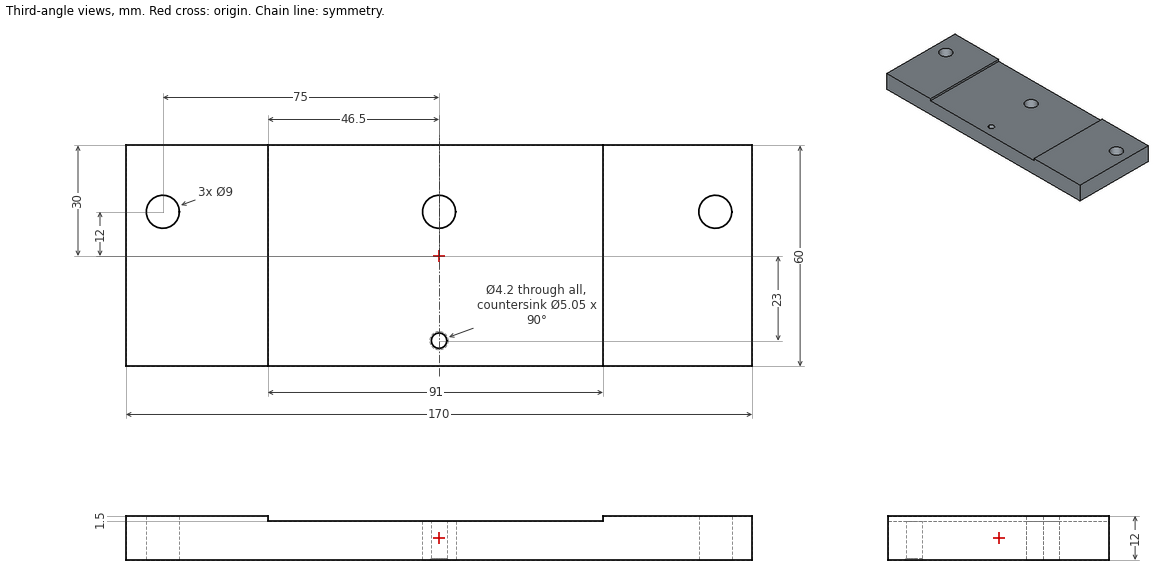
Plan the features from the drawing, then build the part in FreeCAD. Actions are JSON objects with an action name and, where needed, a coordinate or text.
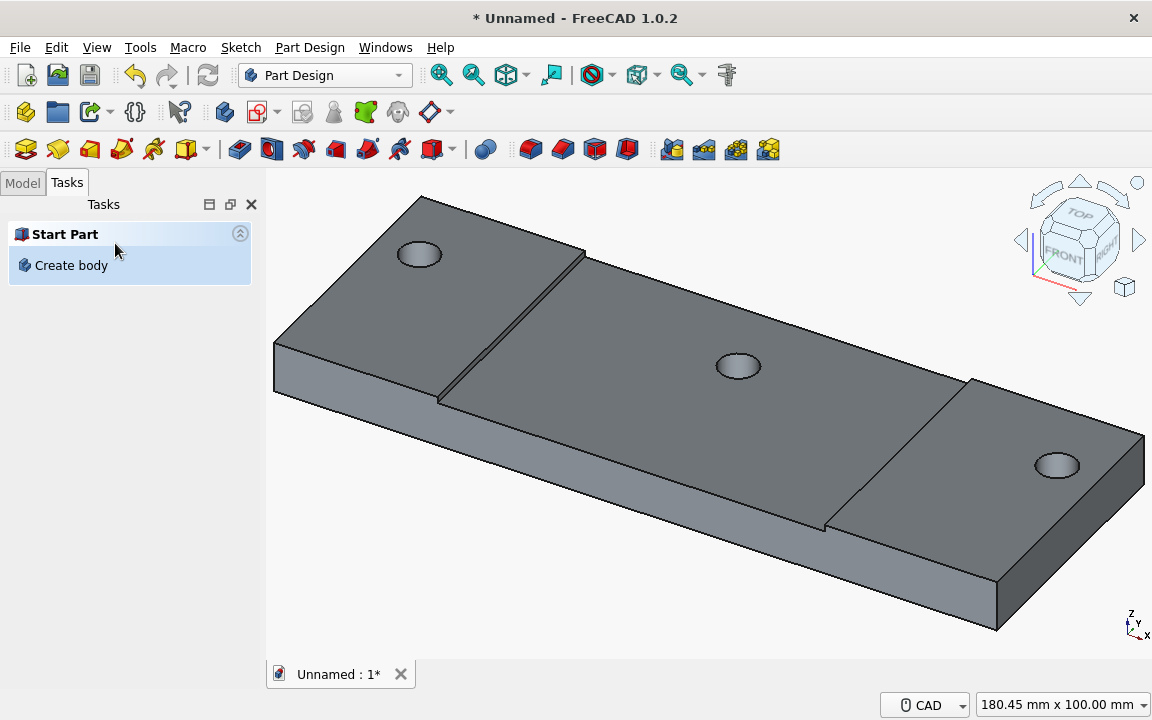
{"action": "key", "text": "5"}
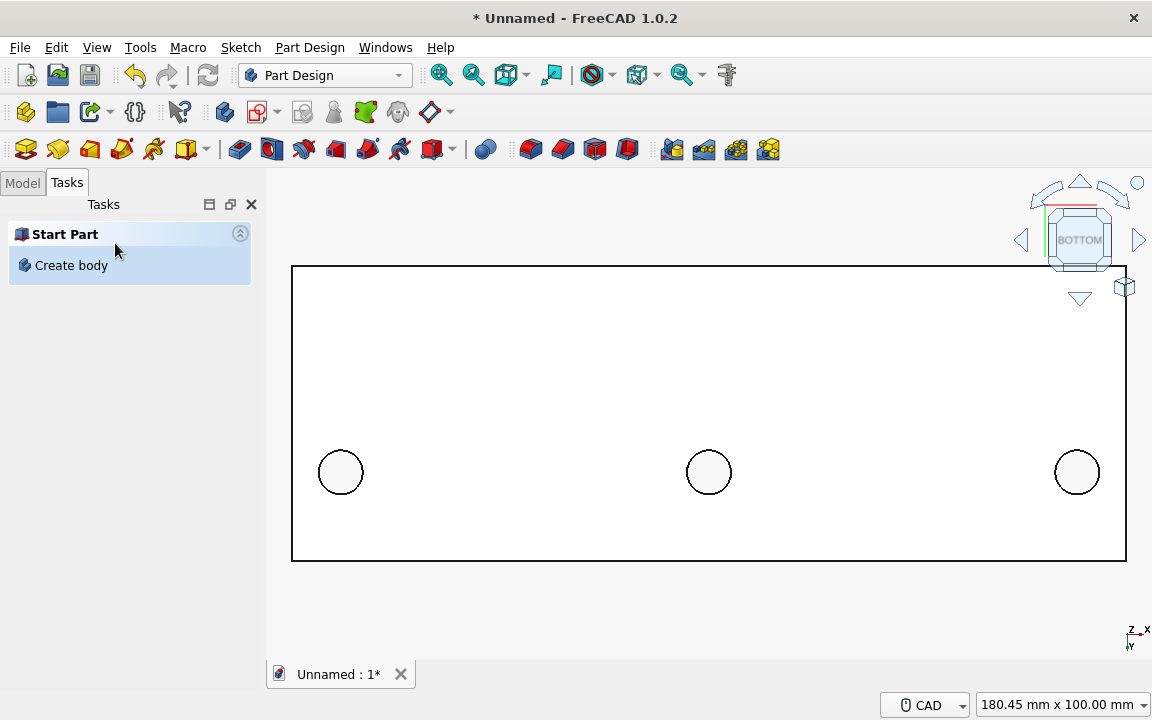
{"action": "left_click", "coordinate": [471, 412]}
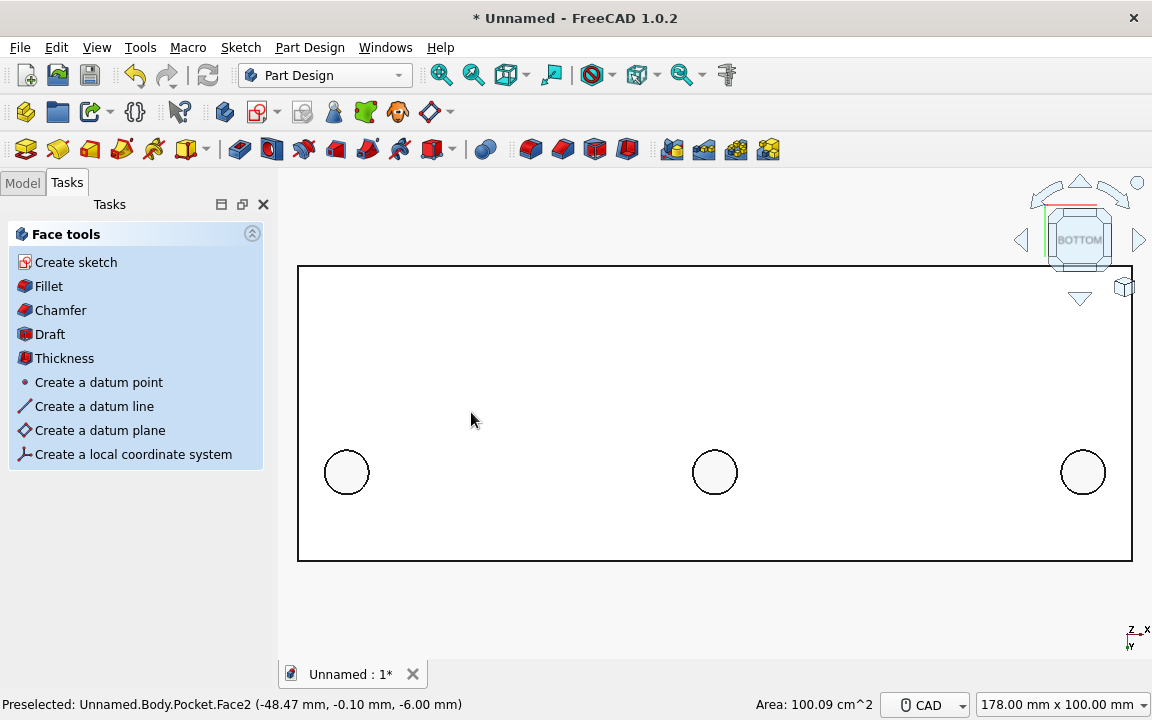
{"action": "left_click", "coordinate": [258, 112]}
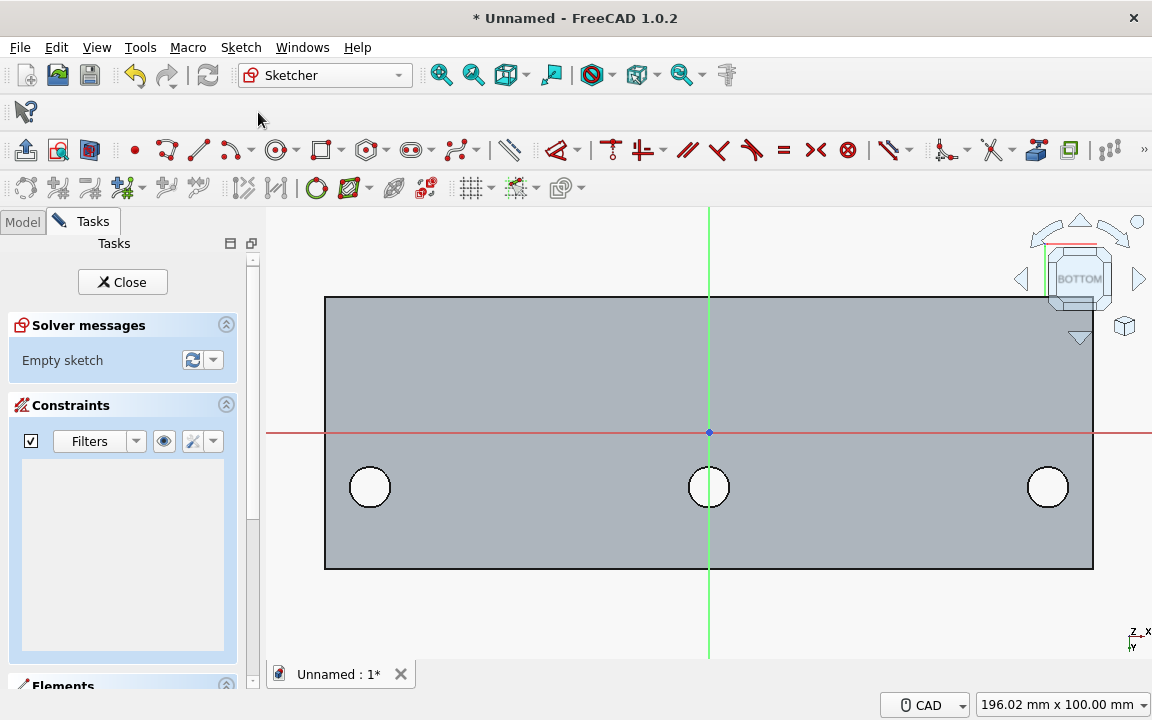
{"action": "scroll", "coordinate": [714, 321], "scroll_direction": "up", "scroll_amount": 13}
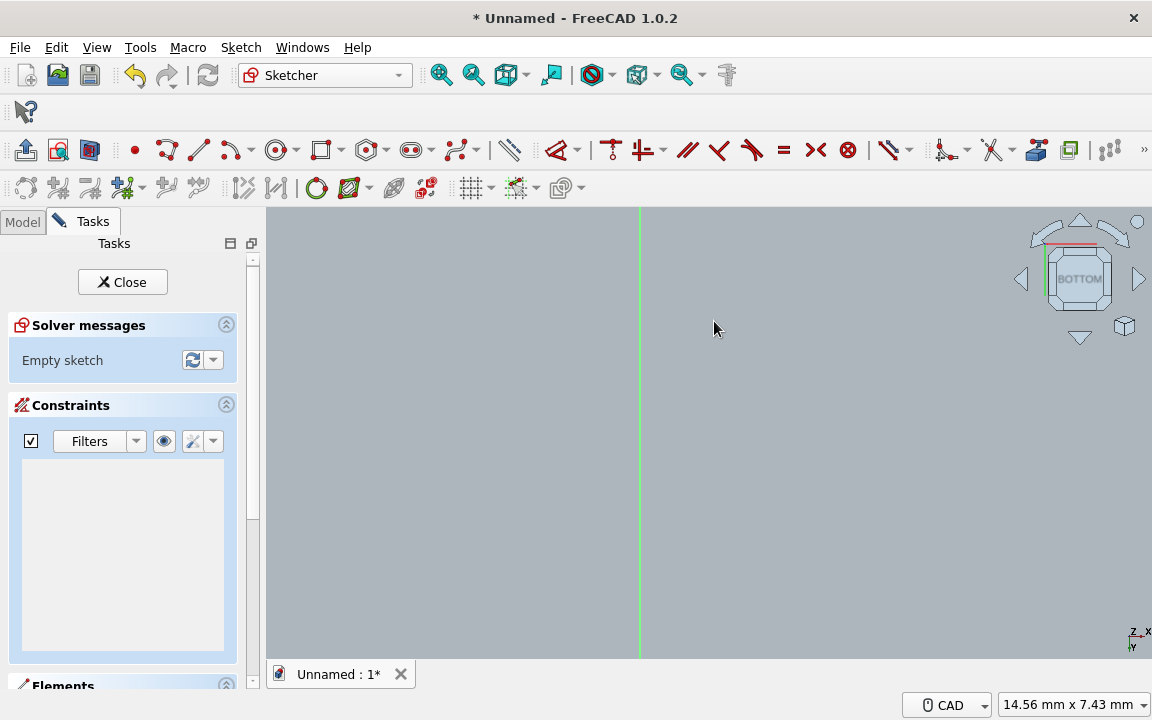
{"action": "key", "text": "g c"}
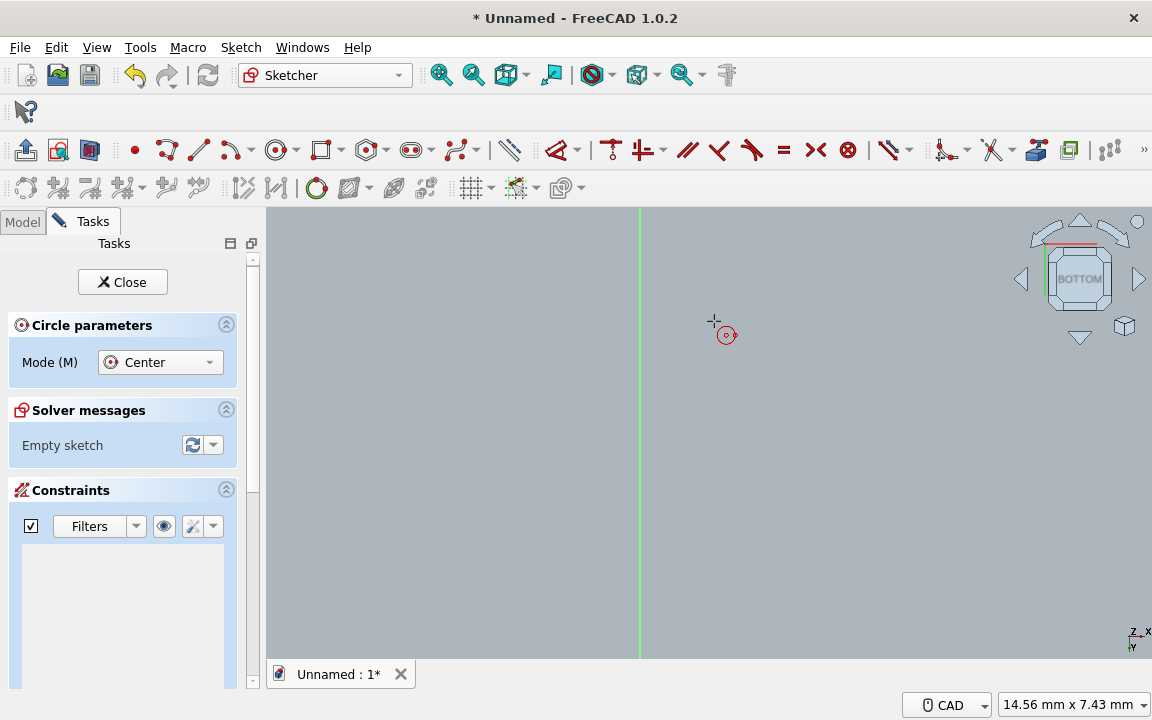
{"action": "left_click", "coordinate": [640, 426]}
{"action": "left_click", "coordinate": [731, 336]}
{"action": "key", "text": "Escape"}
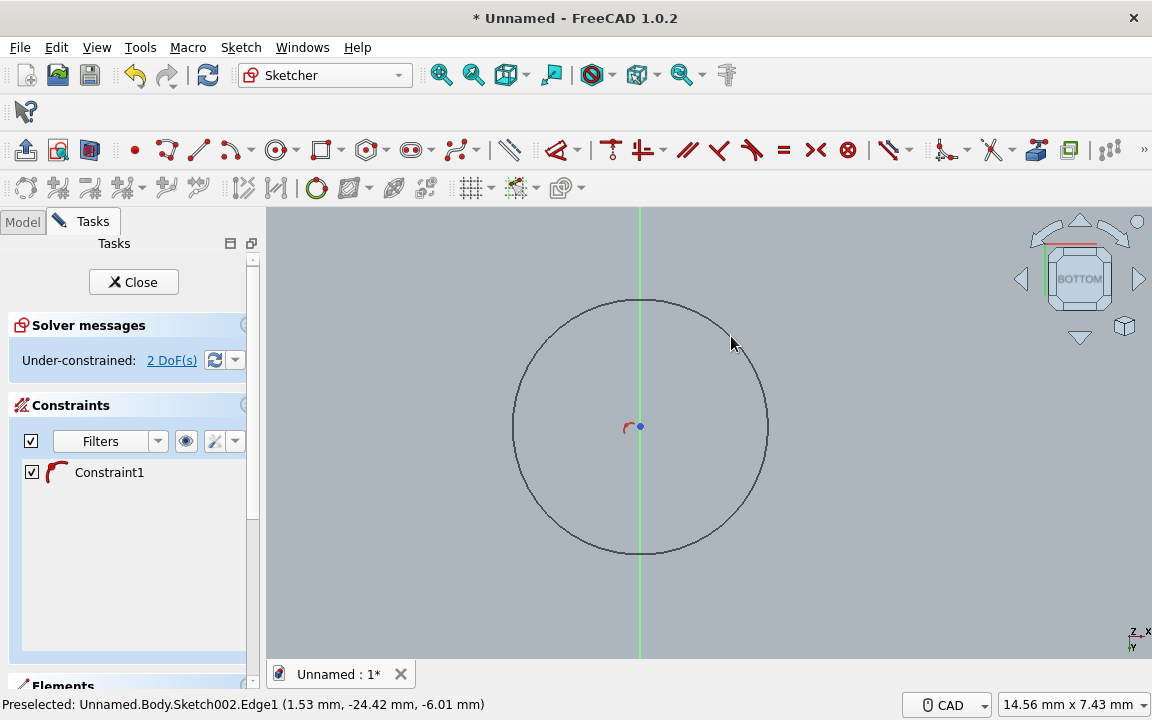
{"action": "key", "text": "d"}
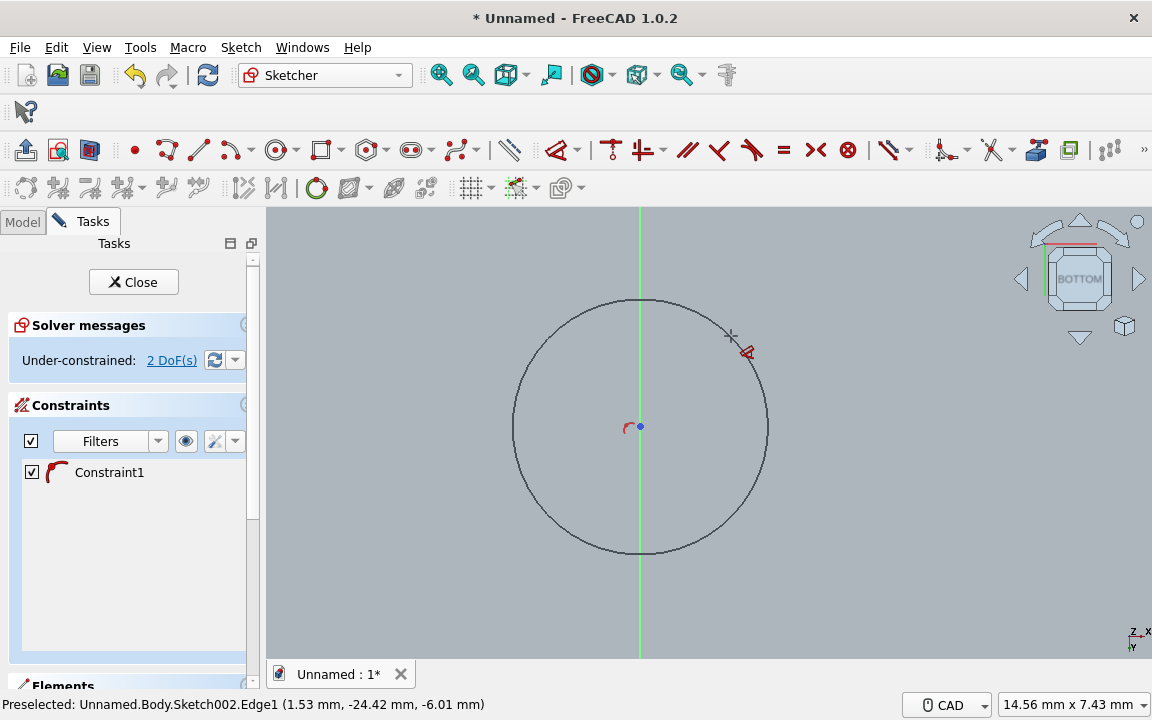
{"action": "left_click", "coordinate": [730, 336]}
{"action": "left_click", "coordinate": [752, 313]}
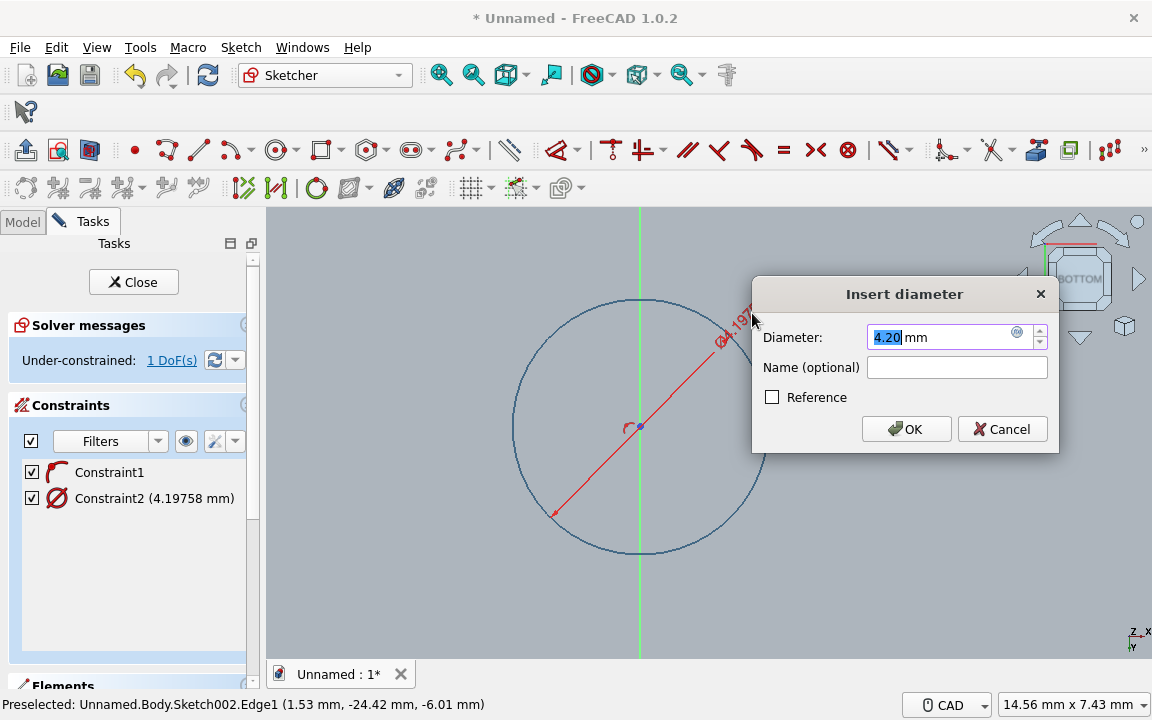
{"action": "type", "text": "4.2"}
{"action": "key", "text": "Return"}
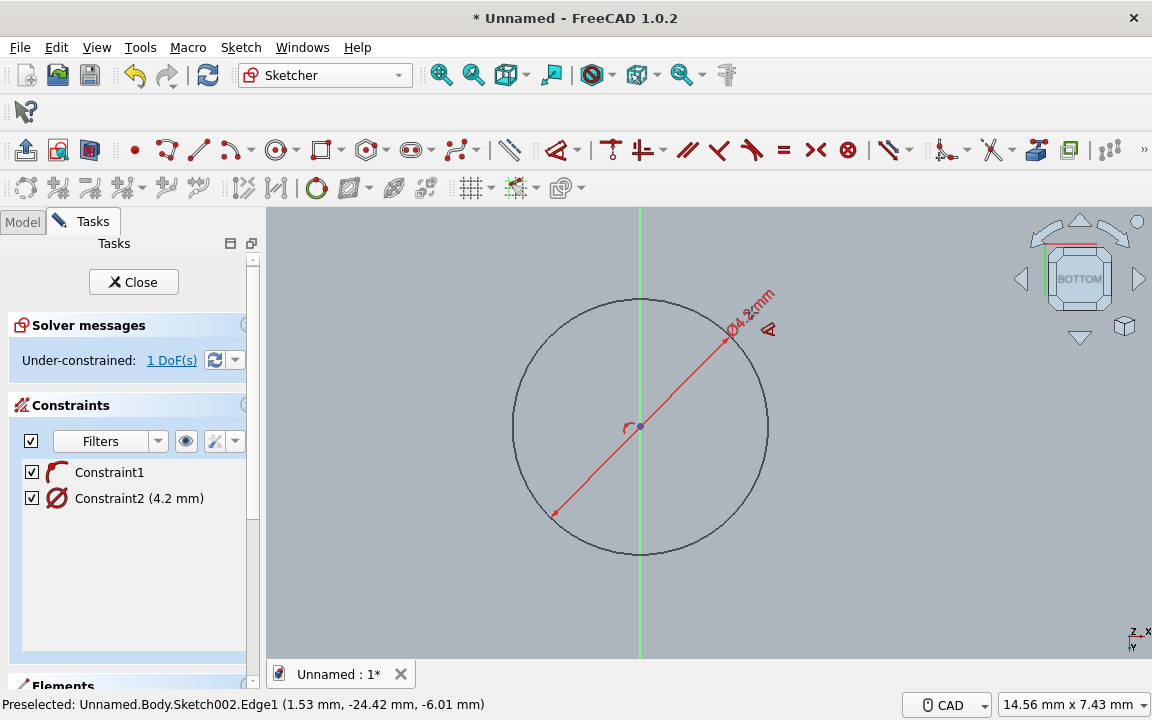
{"action": "left_click", "coordinate": [640, 427]}
{"action": "left_click", "coordinate": [674, 529]}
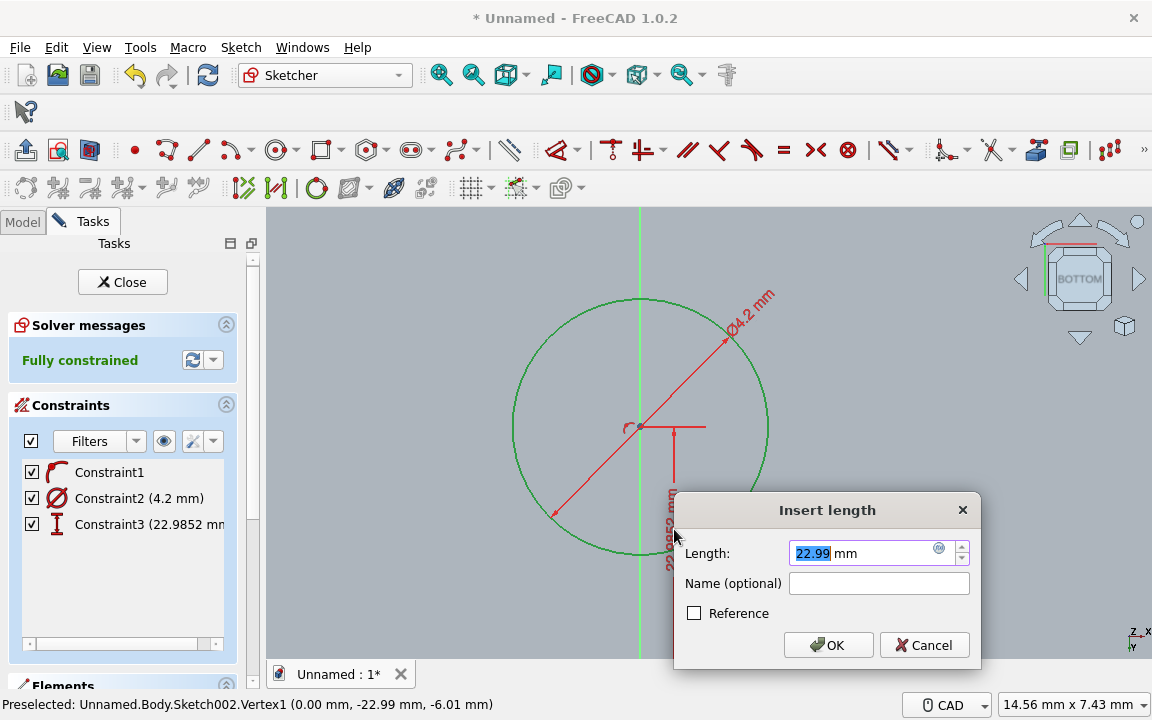
{"action": "type", "text": "23"}
{"action": "key", "text": "Return"}
{"action": "key", "text": "Escape"}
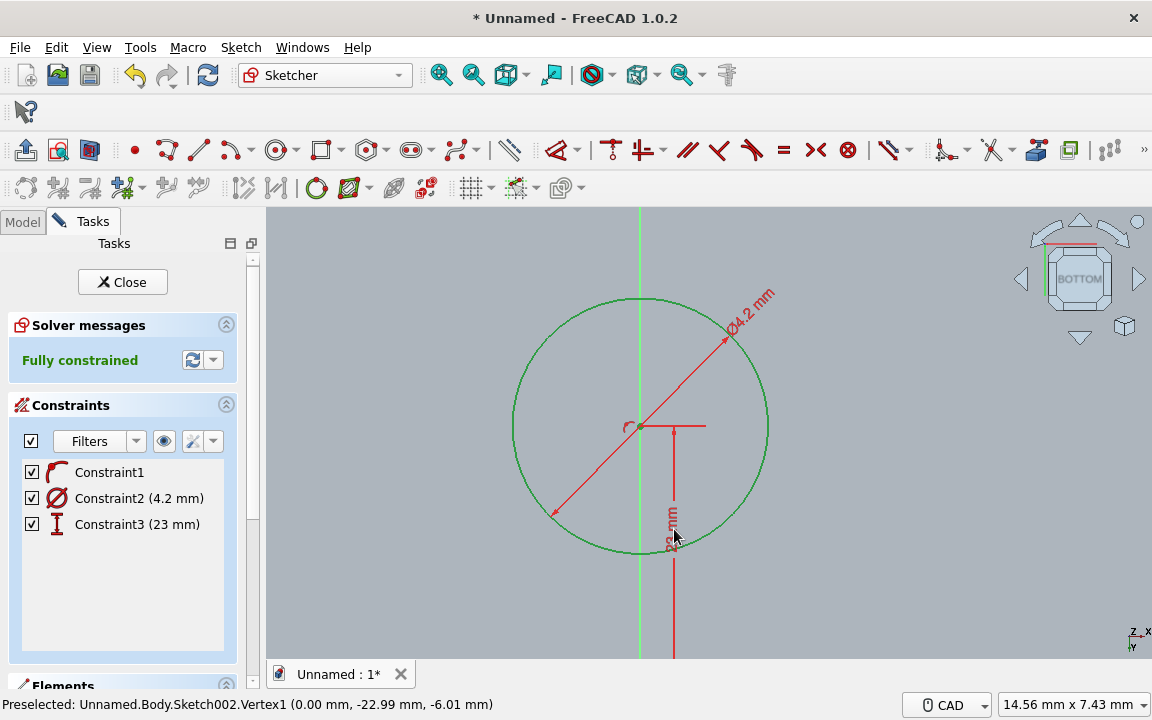
{"action": "left_click", "coordinate": [123, 282]}